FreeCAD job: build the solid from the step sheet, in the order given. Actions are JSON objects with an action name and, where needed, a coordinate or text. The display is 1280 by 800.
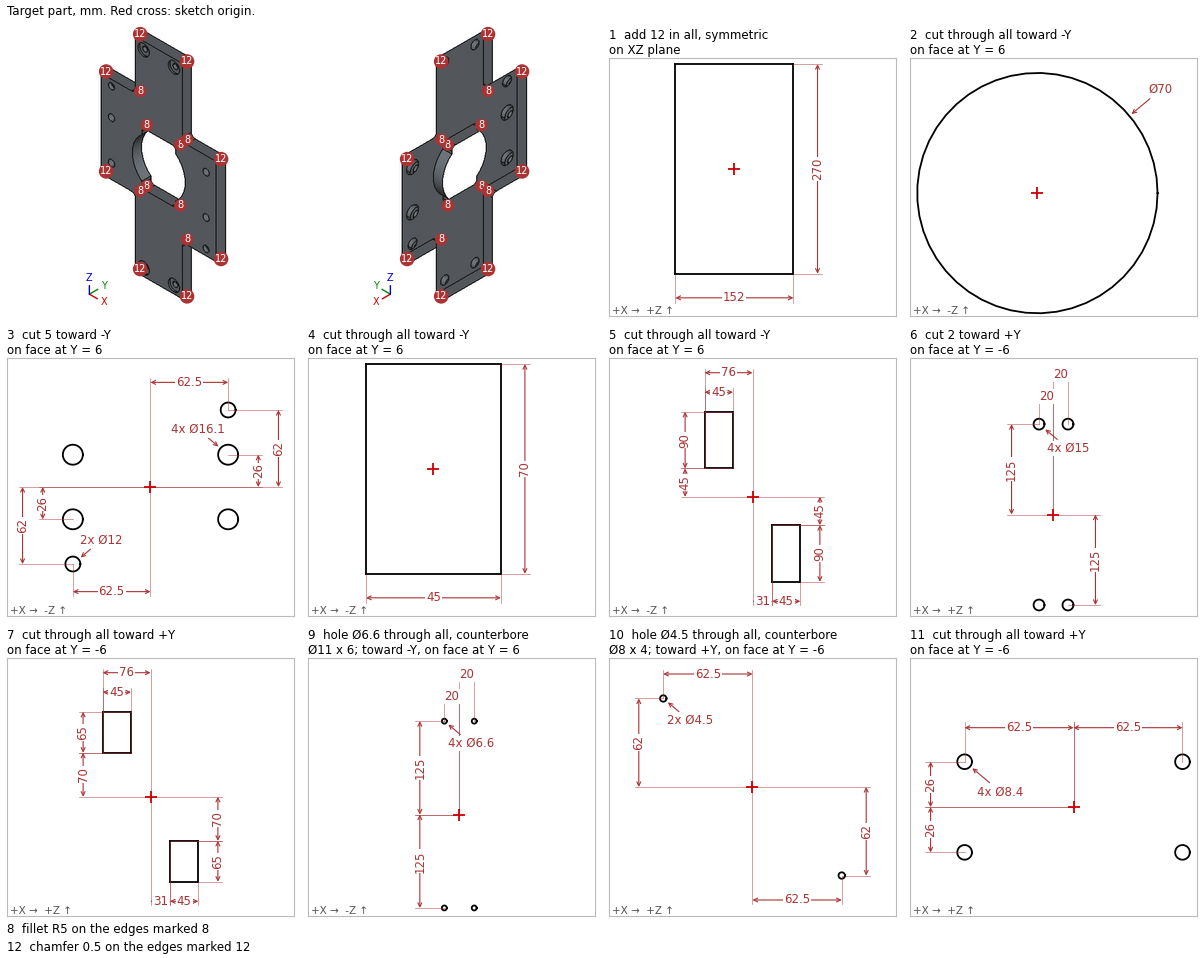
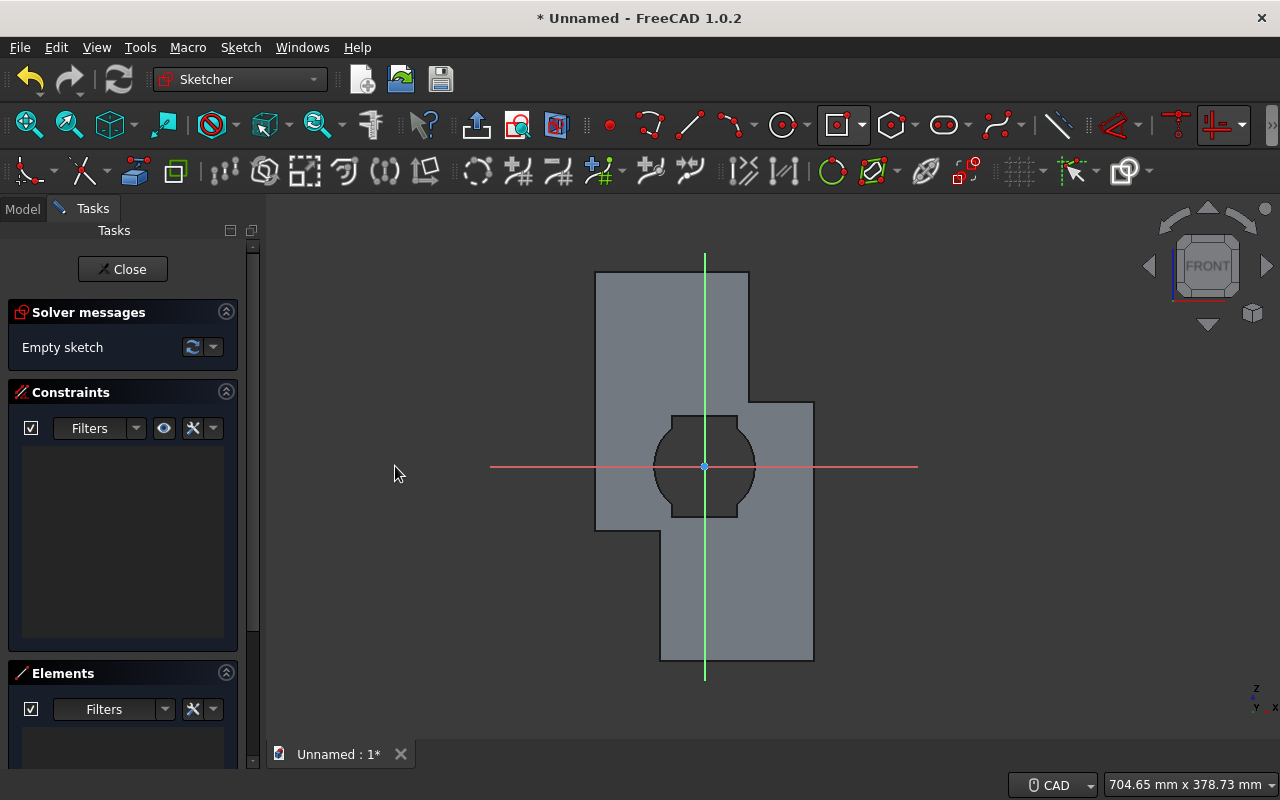
{"action": "key", "text": "g c"}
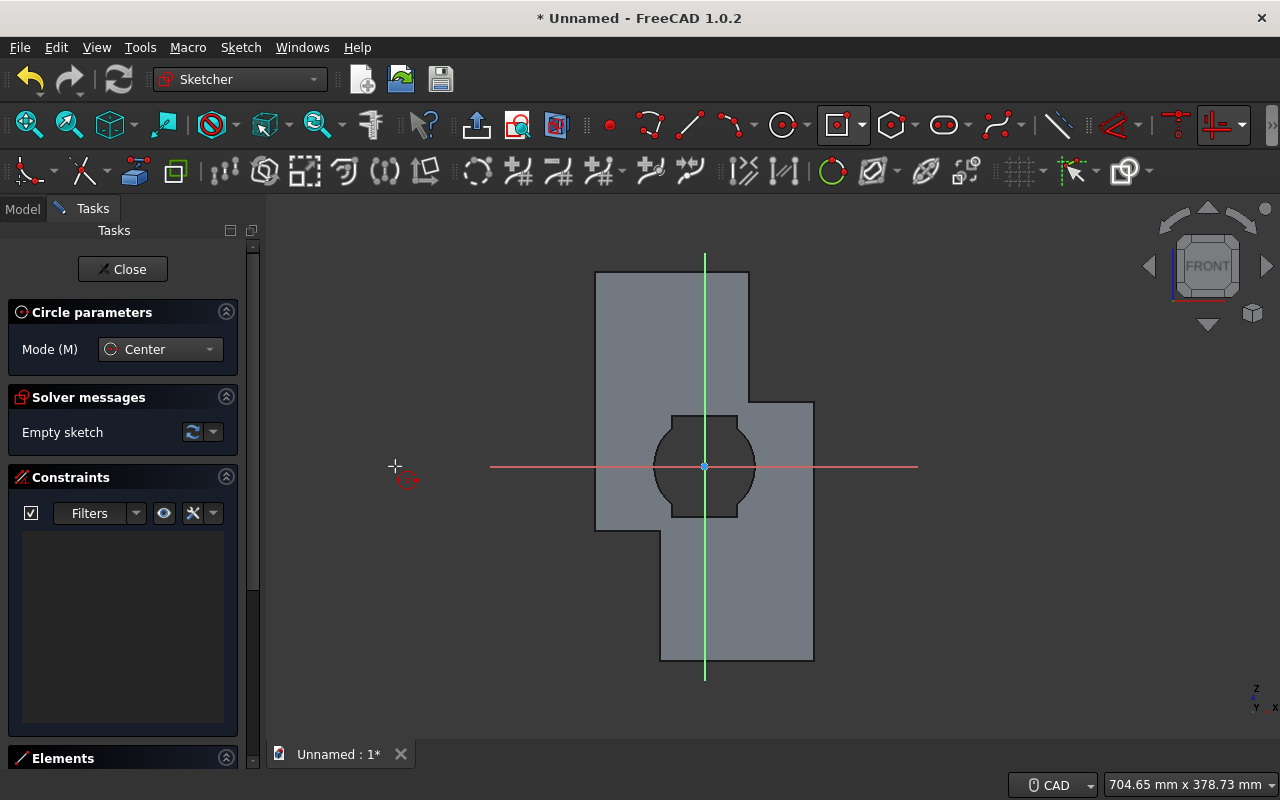
{"action": "scroll", "coordinate": [676, 287], "scroll_direction": "up", "scroll_amount": 4}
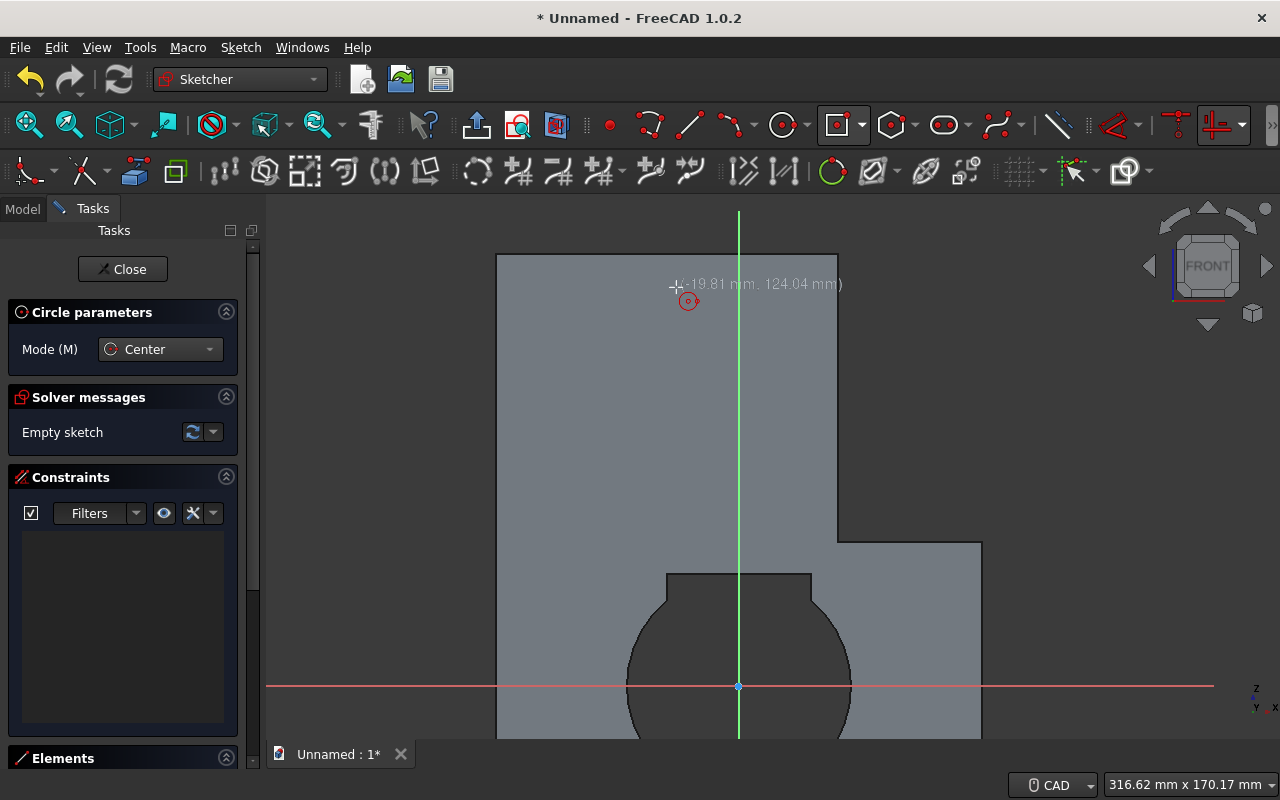
{"action": "left_click", "coordinate": [675, 286]}
{"action": "mouse_move", "coordinate": [692, 269]}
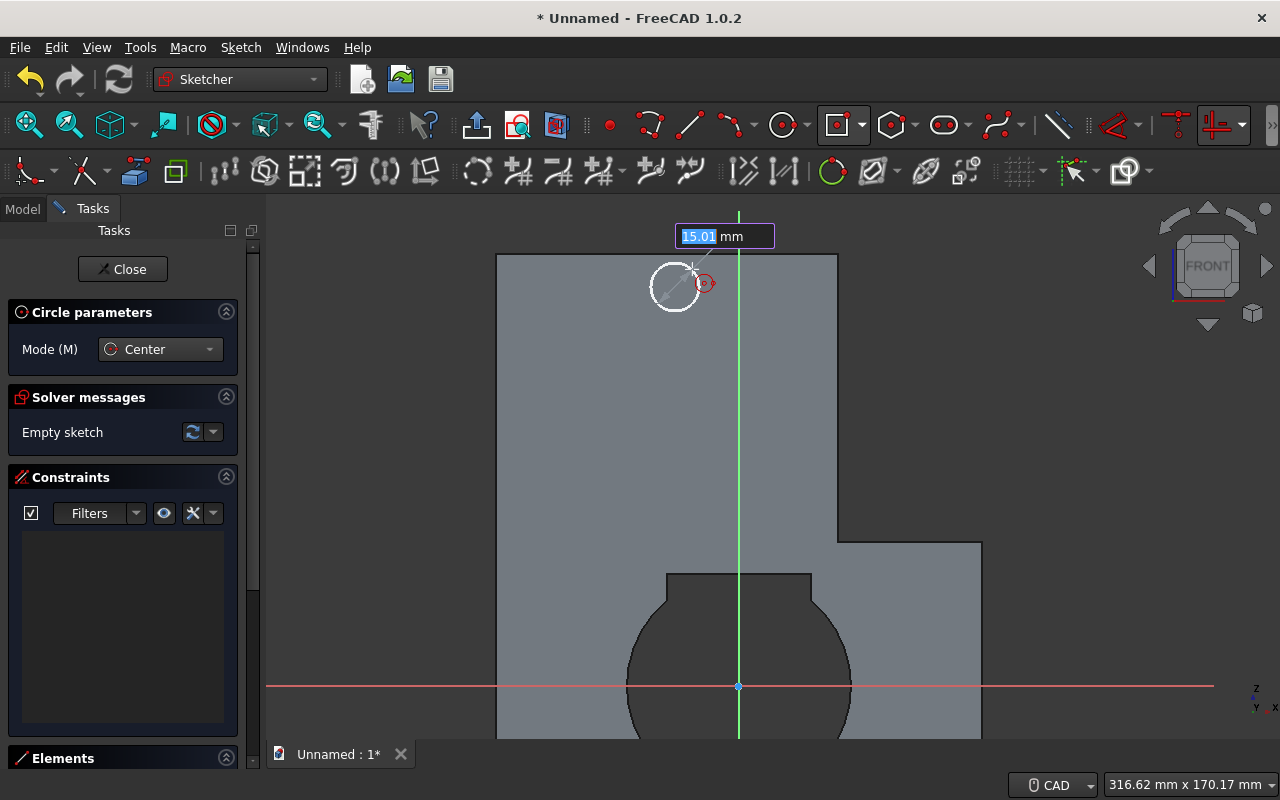
{"action": "type", "text": "15"}
{"action": "key", "text": "Return"}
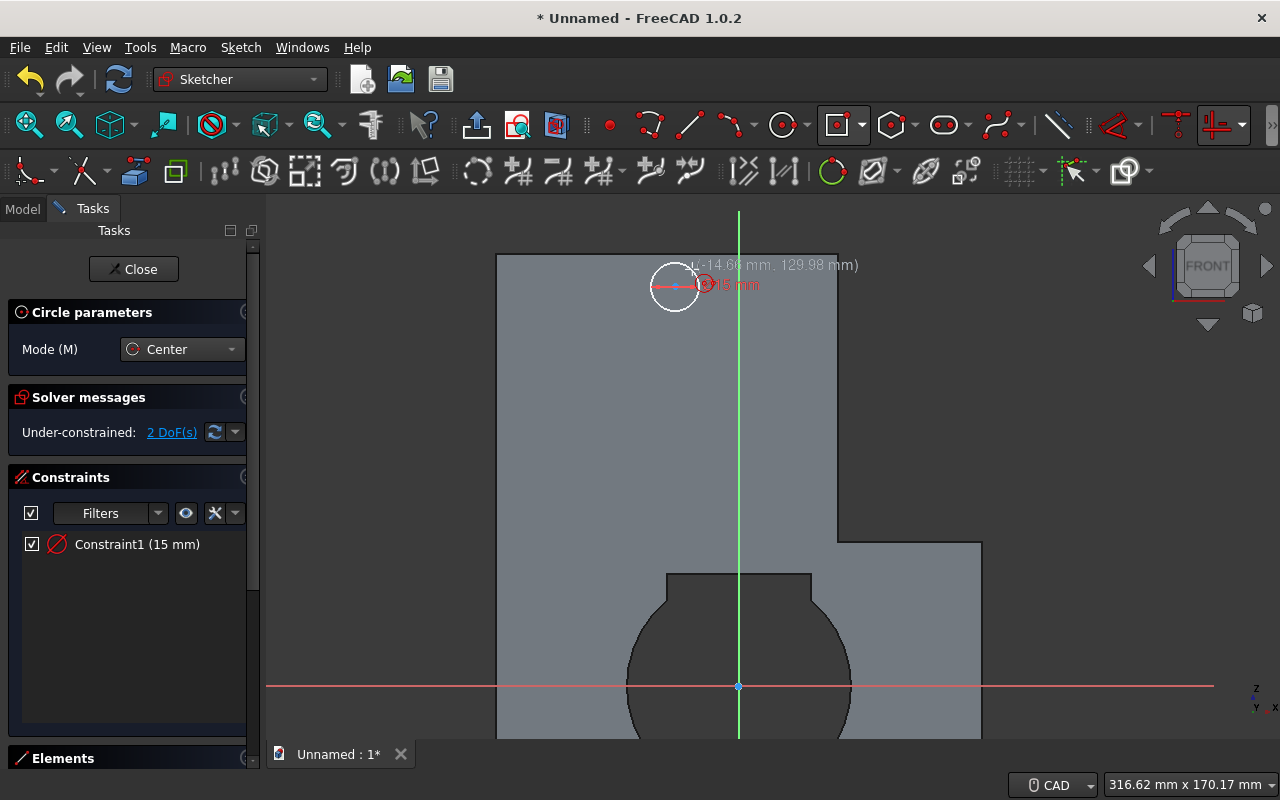
{"action": "left_click", "coordinate": [803, 286]}
{"action": "mouse_move", "coordinate": [820, 269]}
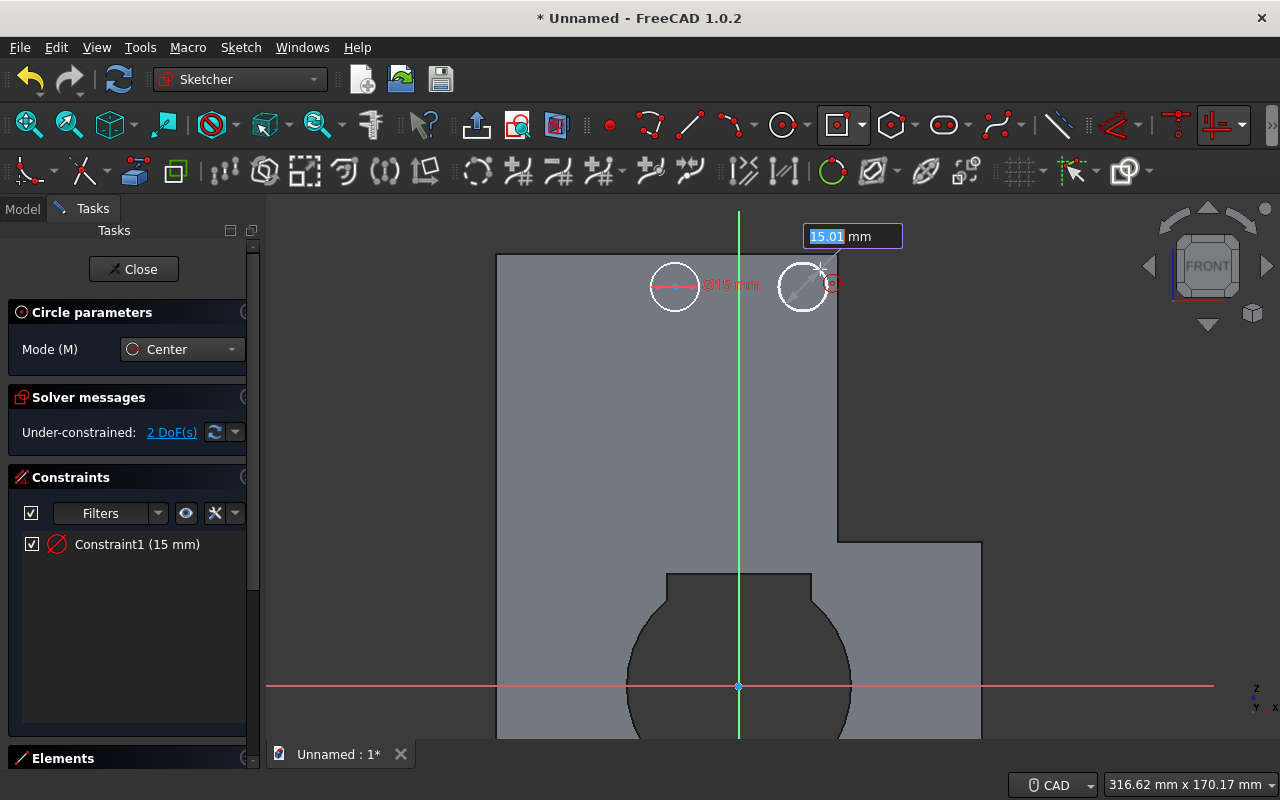
{"action": "type", "text": "15"}
{"action": "key", "text": "Return"}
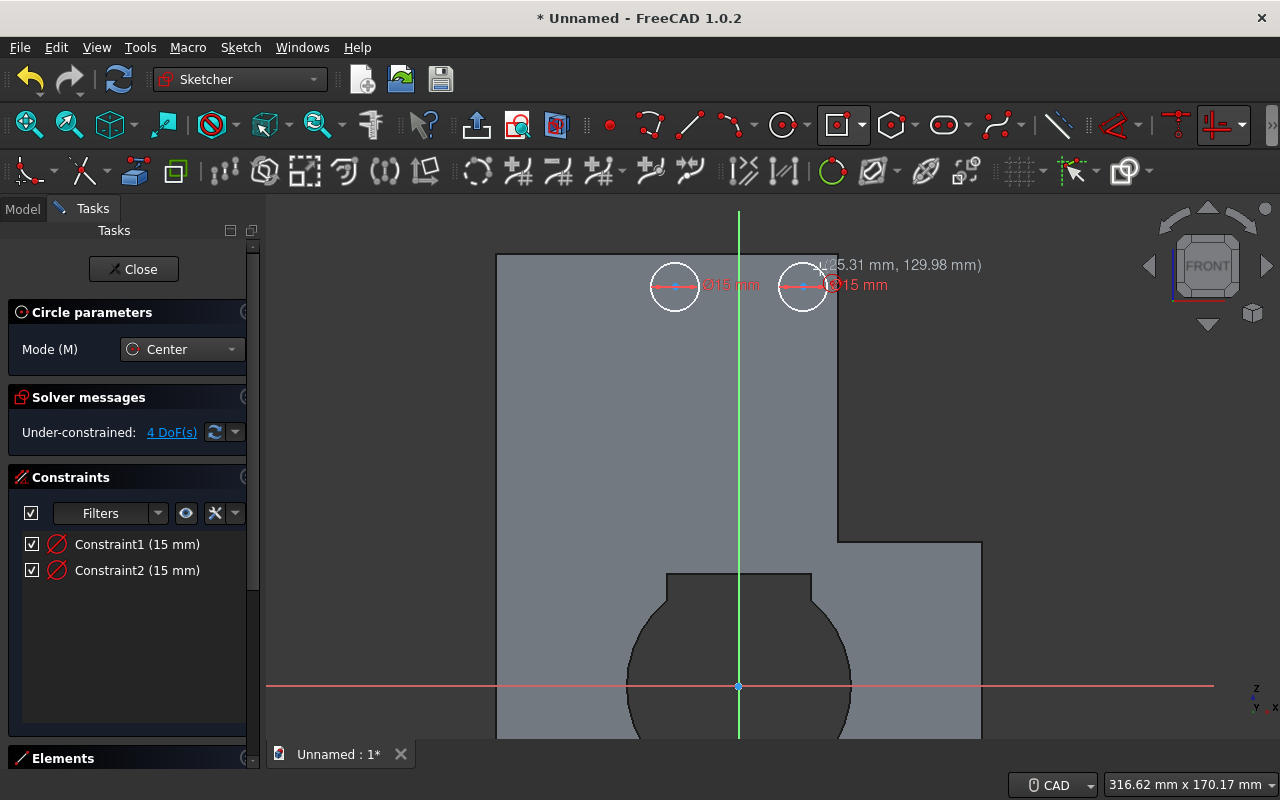
{"action": "scroll", "coordinate": [676, 287], "scroll_direction": "down", "scroll_amount": 4}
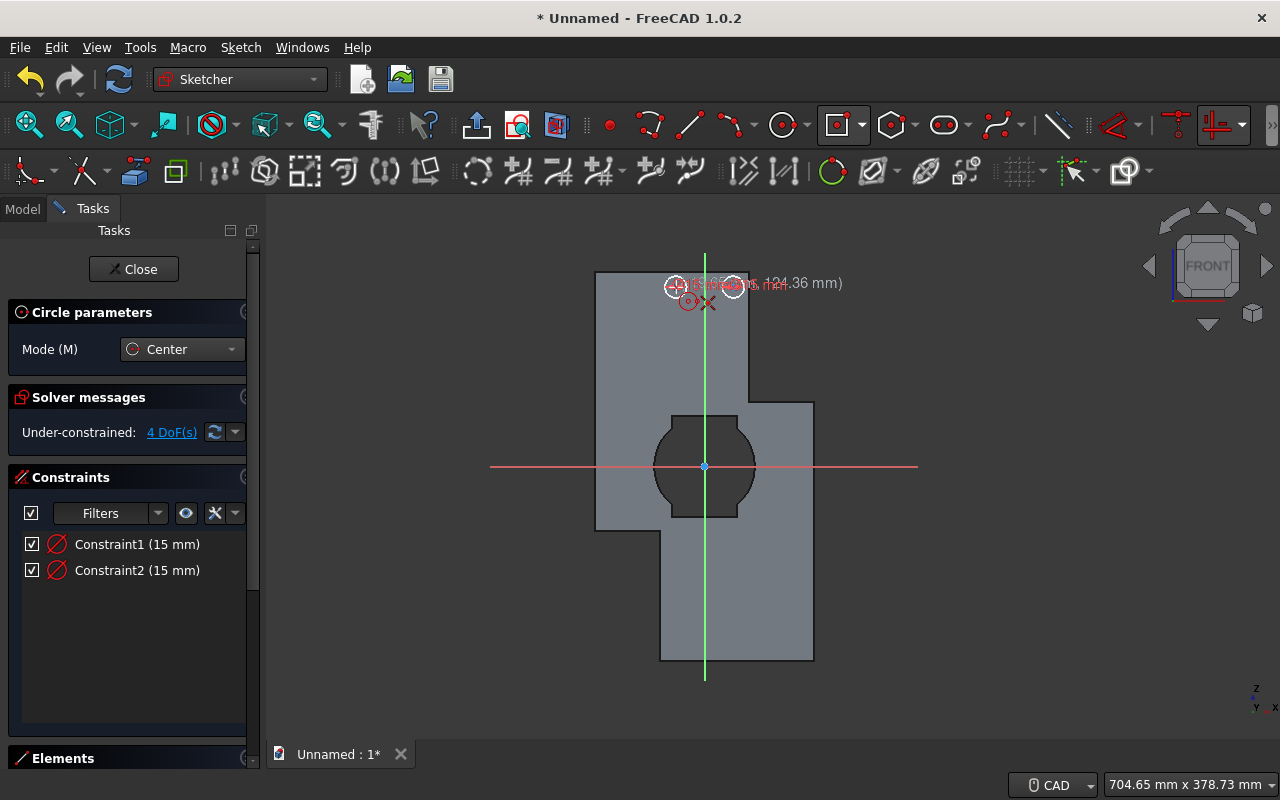
{"action": "scroll", "coordinate": [733, 646], "scroll_direction": "up", "scroll_amount": 4}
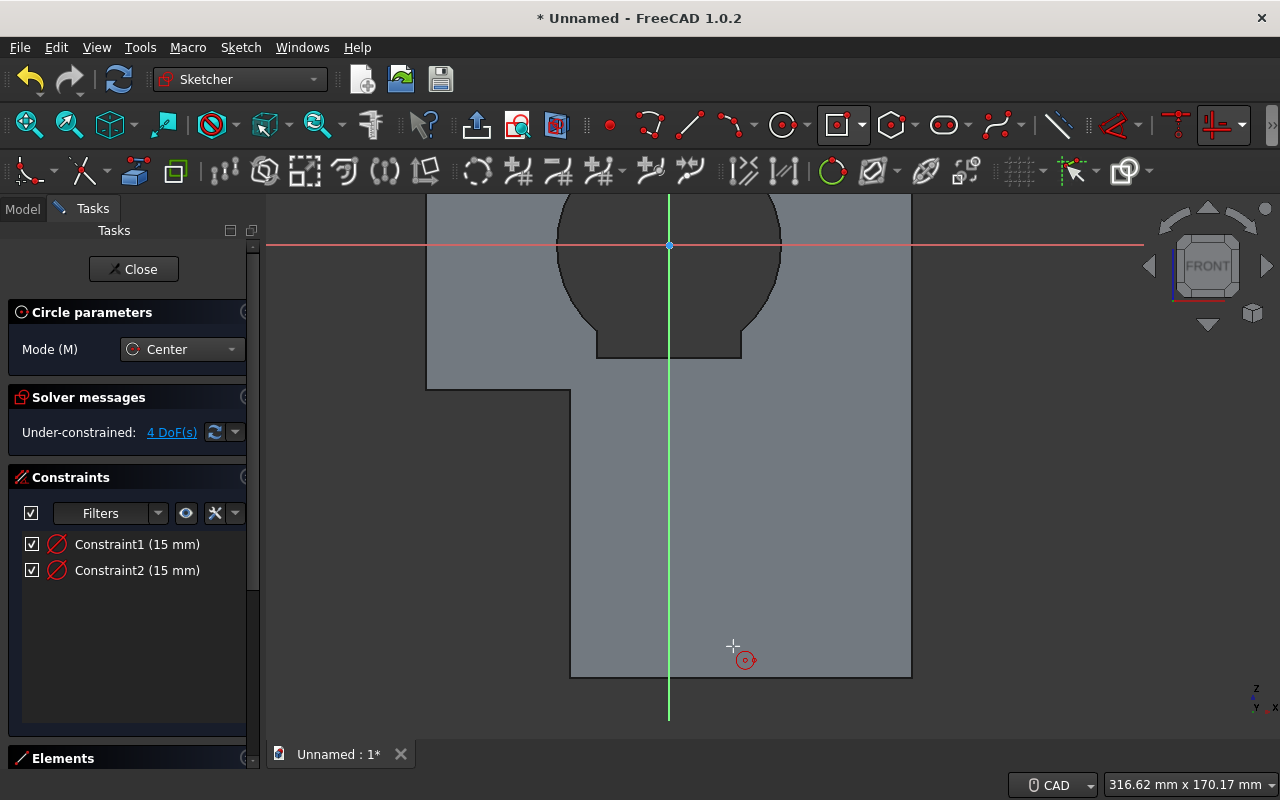
{"action": "left_click", "coordinate": [733, 646]}
{"action": "mouse_move", "coordinate": [750, 629]}